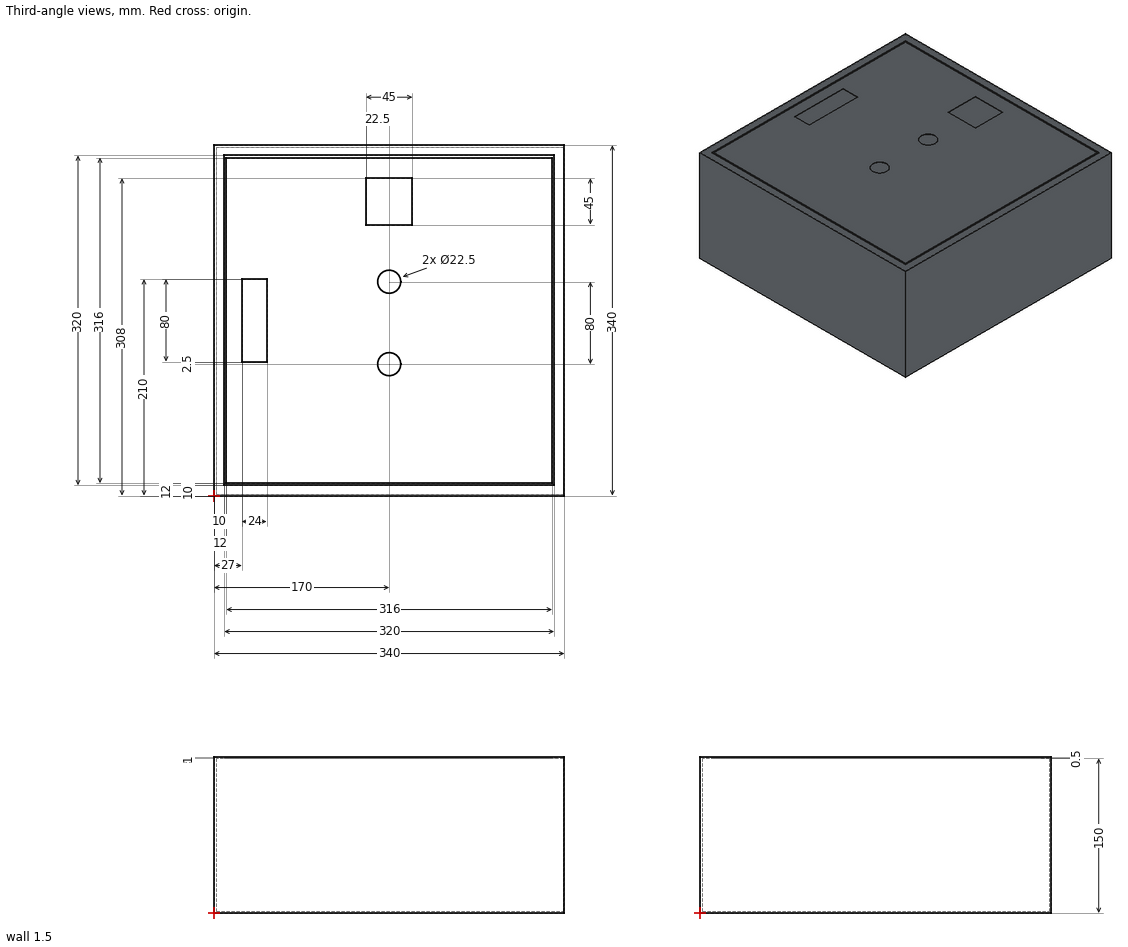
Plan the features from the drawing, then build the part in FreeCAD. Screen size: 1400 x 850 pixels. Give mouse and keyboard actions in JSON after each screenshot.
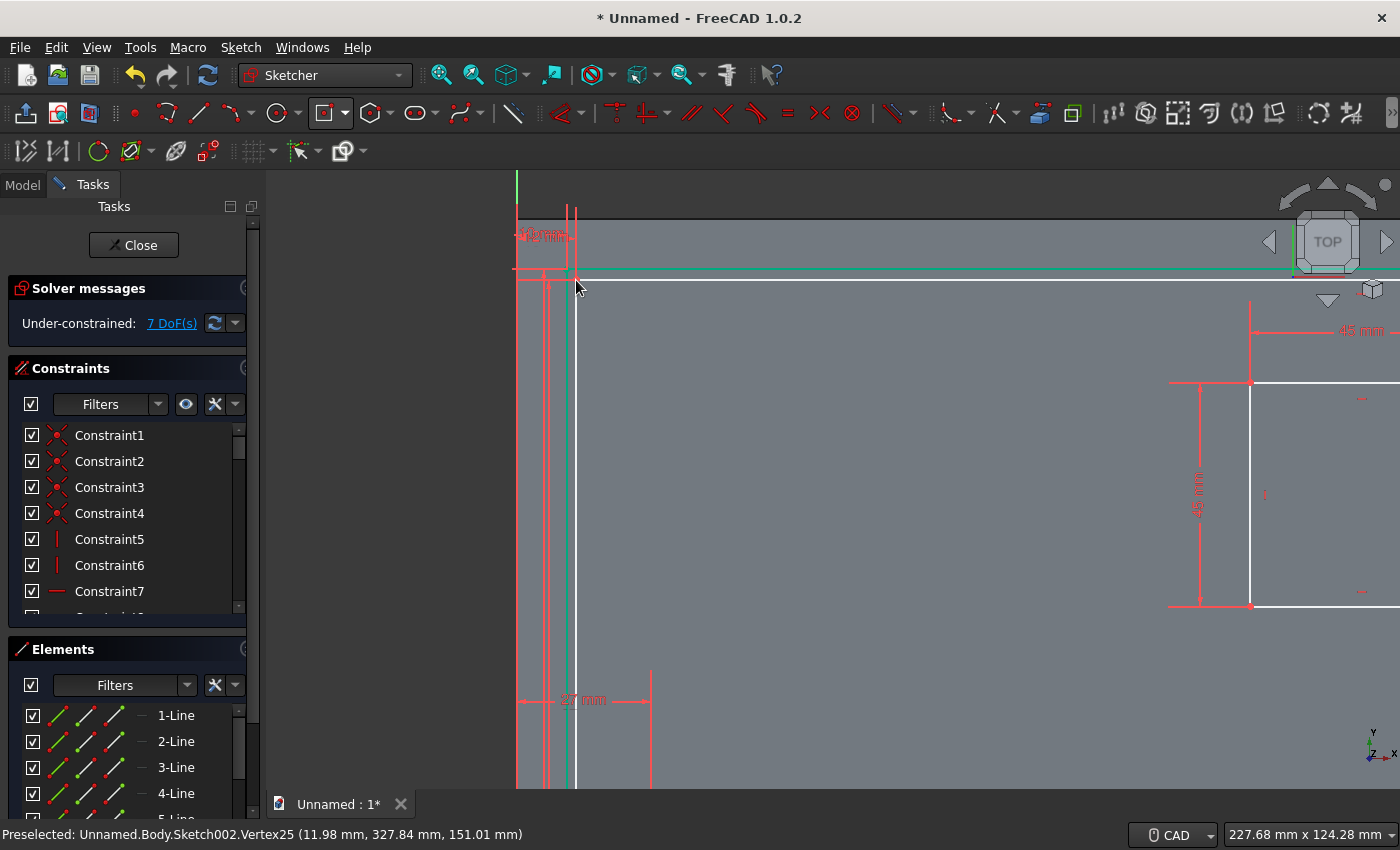
{"action": "scroll", "coordinate": [577, 279], "scroll_direction": "down", "scroll_amount": 7}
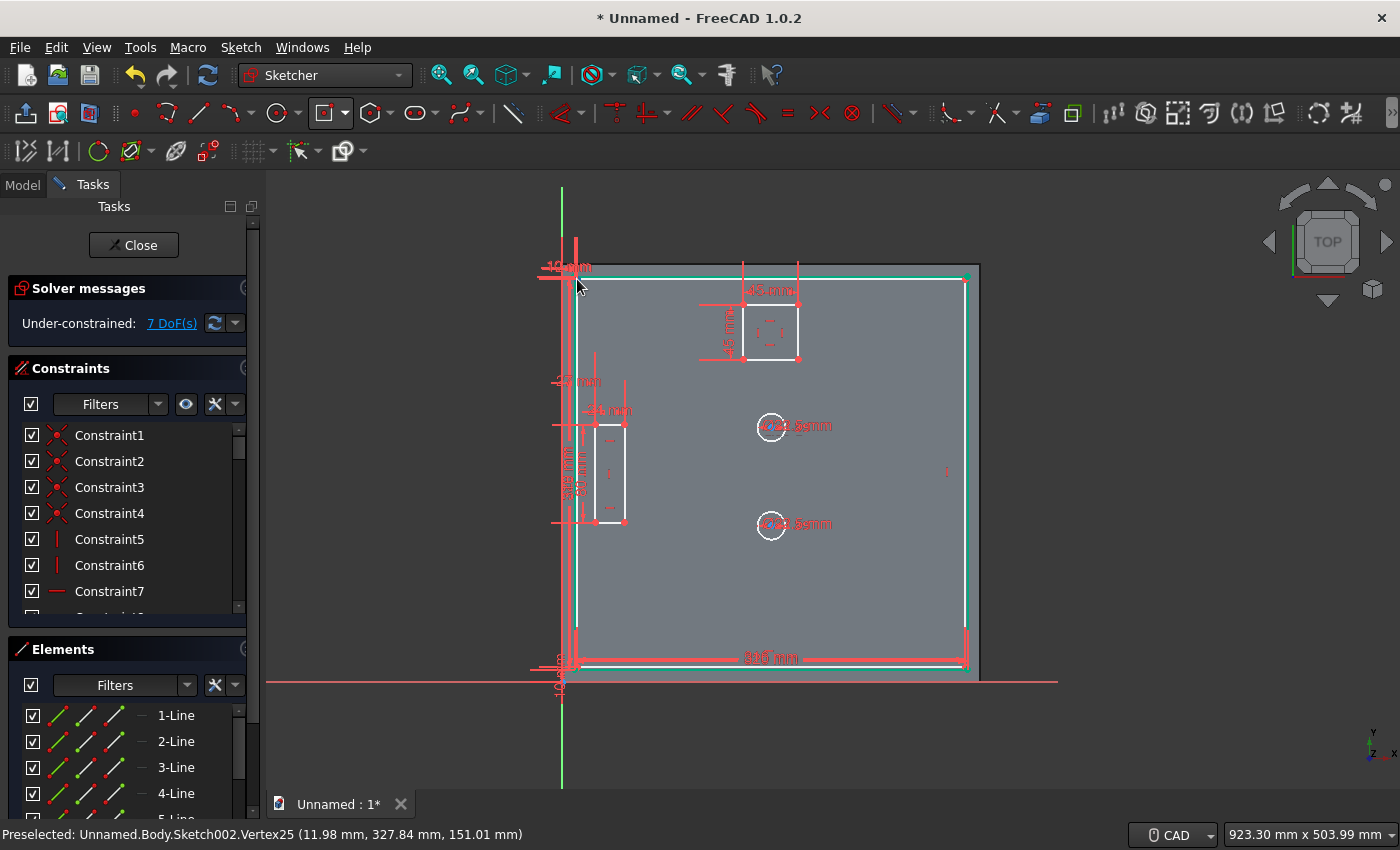
{"action": "scroll", "coordinate": [577, 667], "scroll_direction": "up", "scroll_amount": 7}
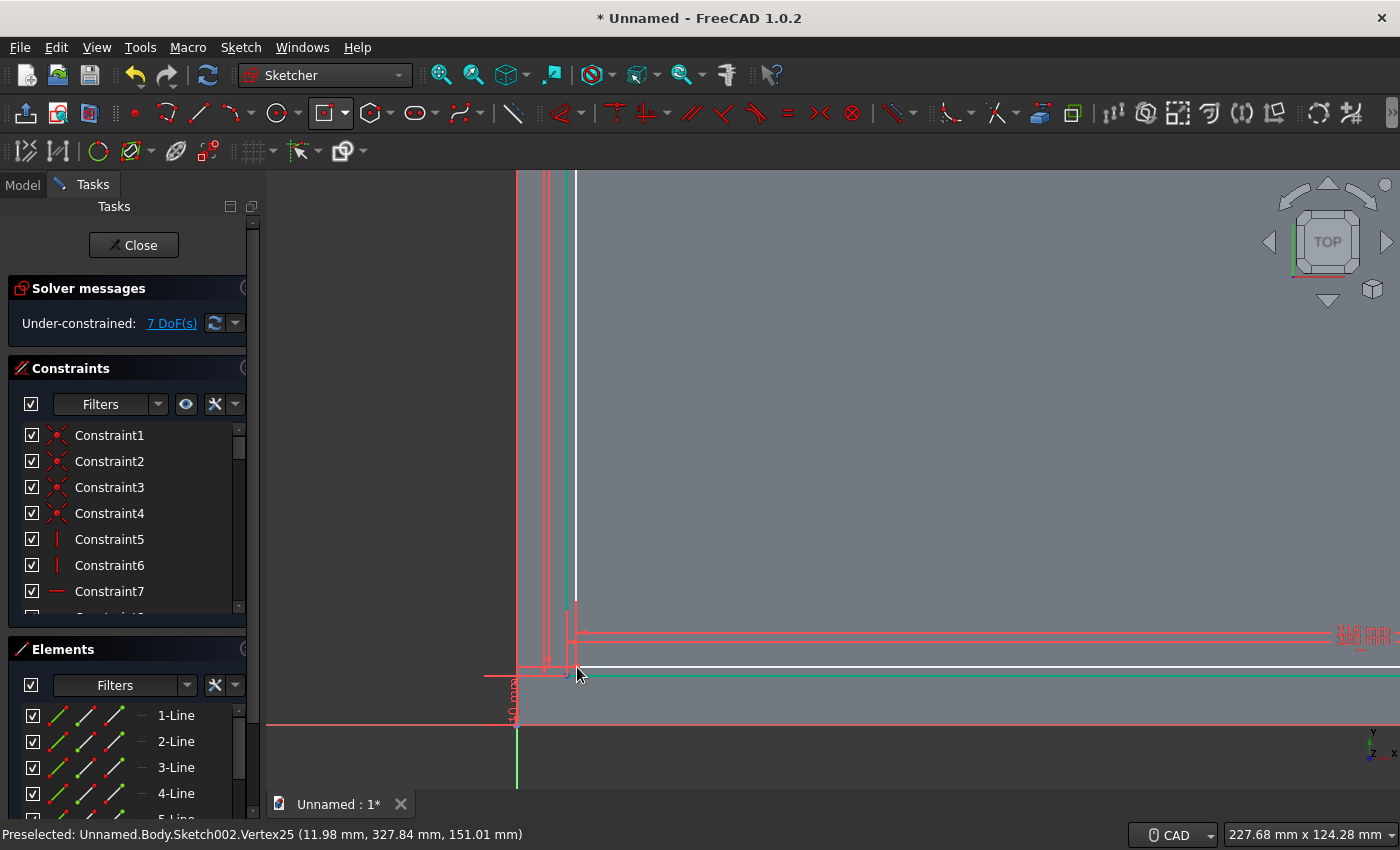
{"action": "left_click", "coordinate": [576, 667]}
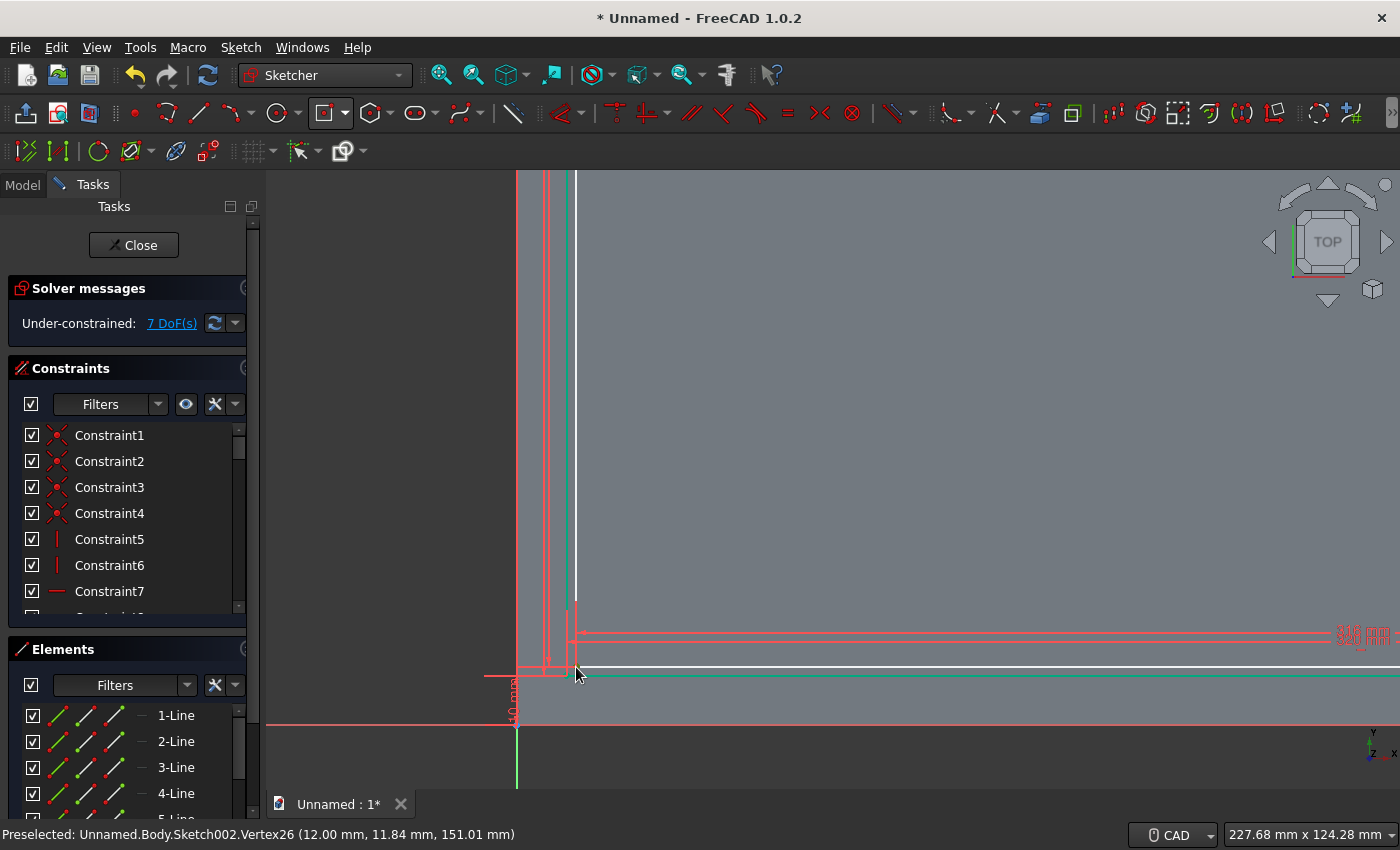
{"action": "key", "text": "i"}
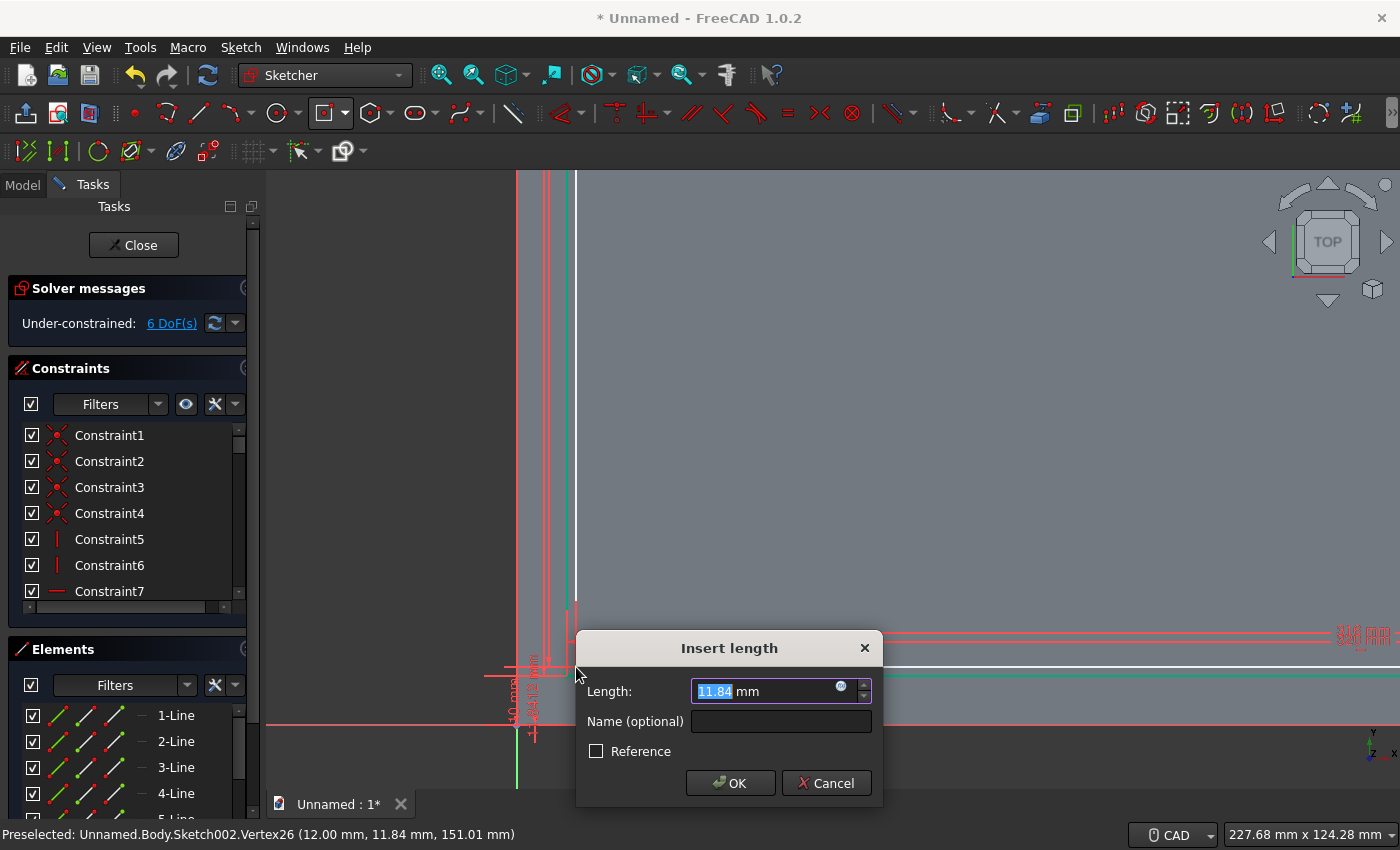
{"action": "type", "text": "12"}
{"action": "key", "text": "Return"}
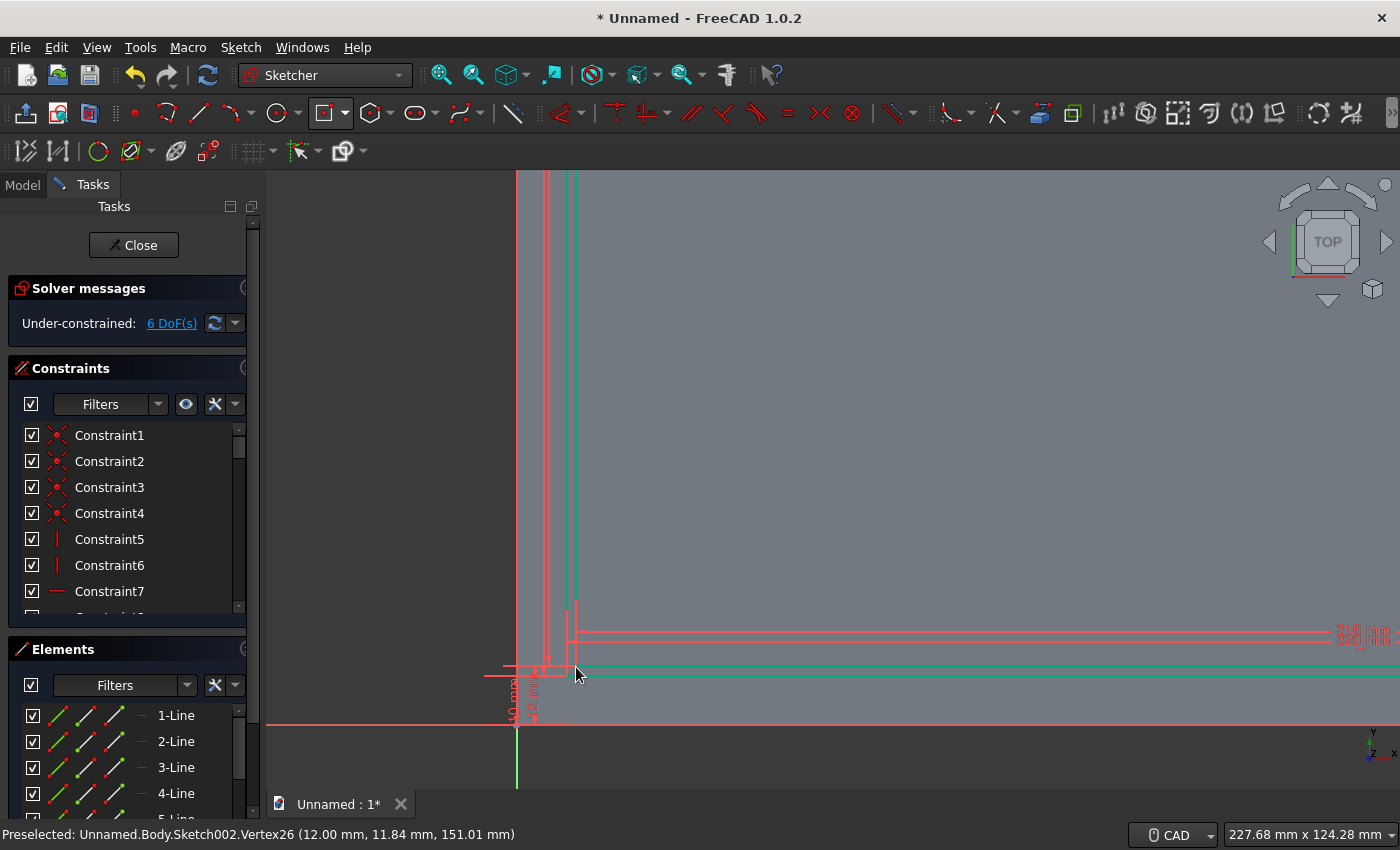
{"action": "scroll", "coordinate": [577, 668], "scroll_direction": "down", "scroll_amount": 7}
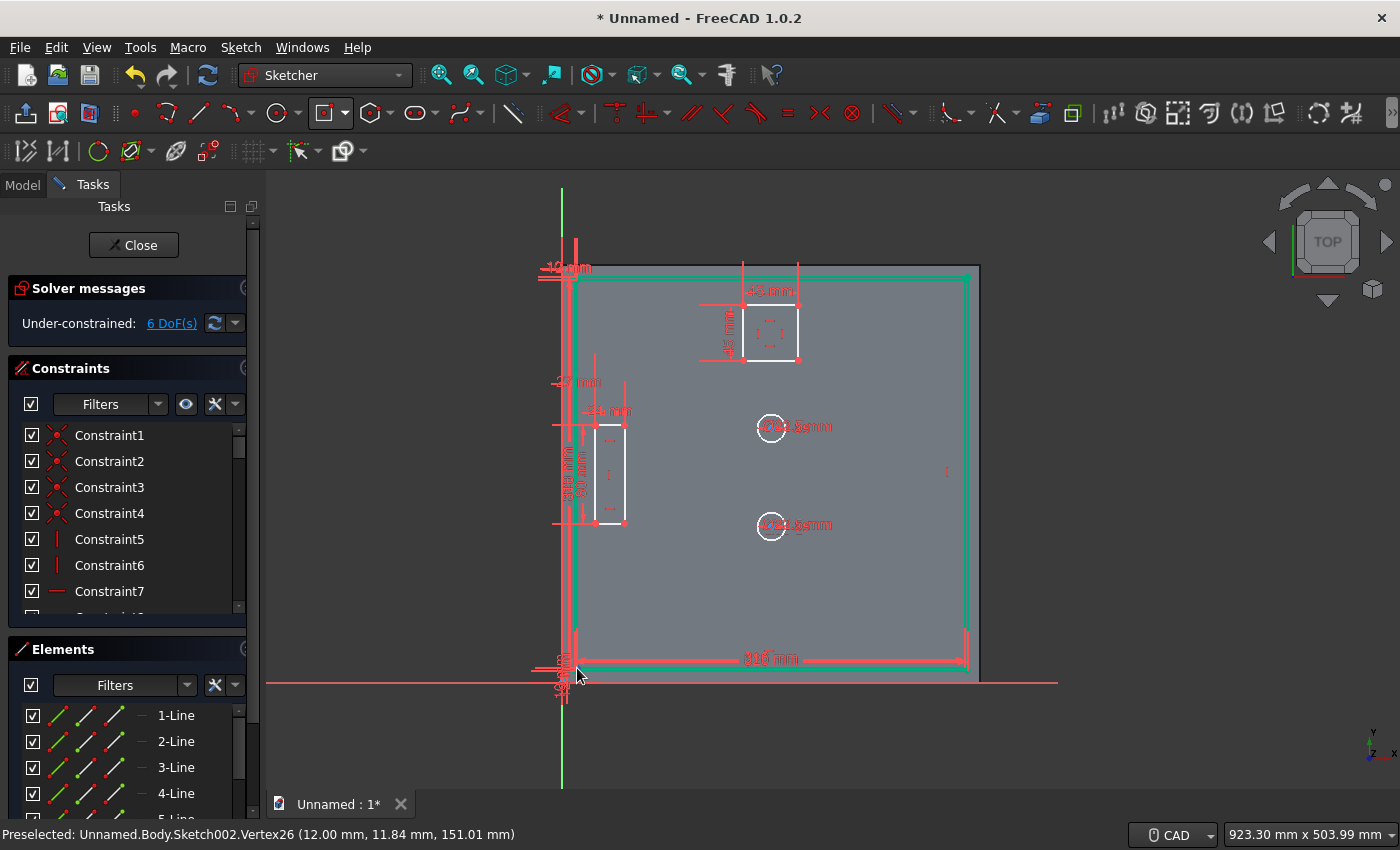
{"action": "left_click", "coordinate": [771, 428]}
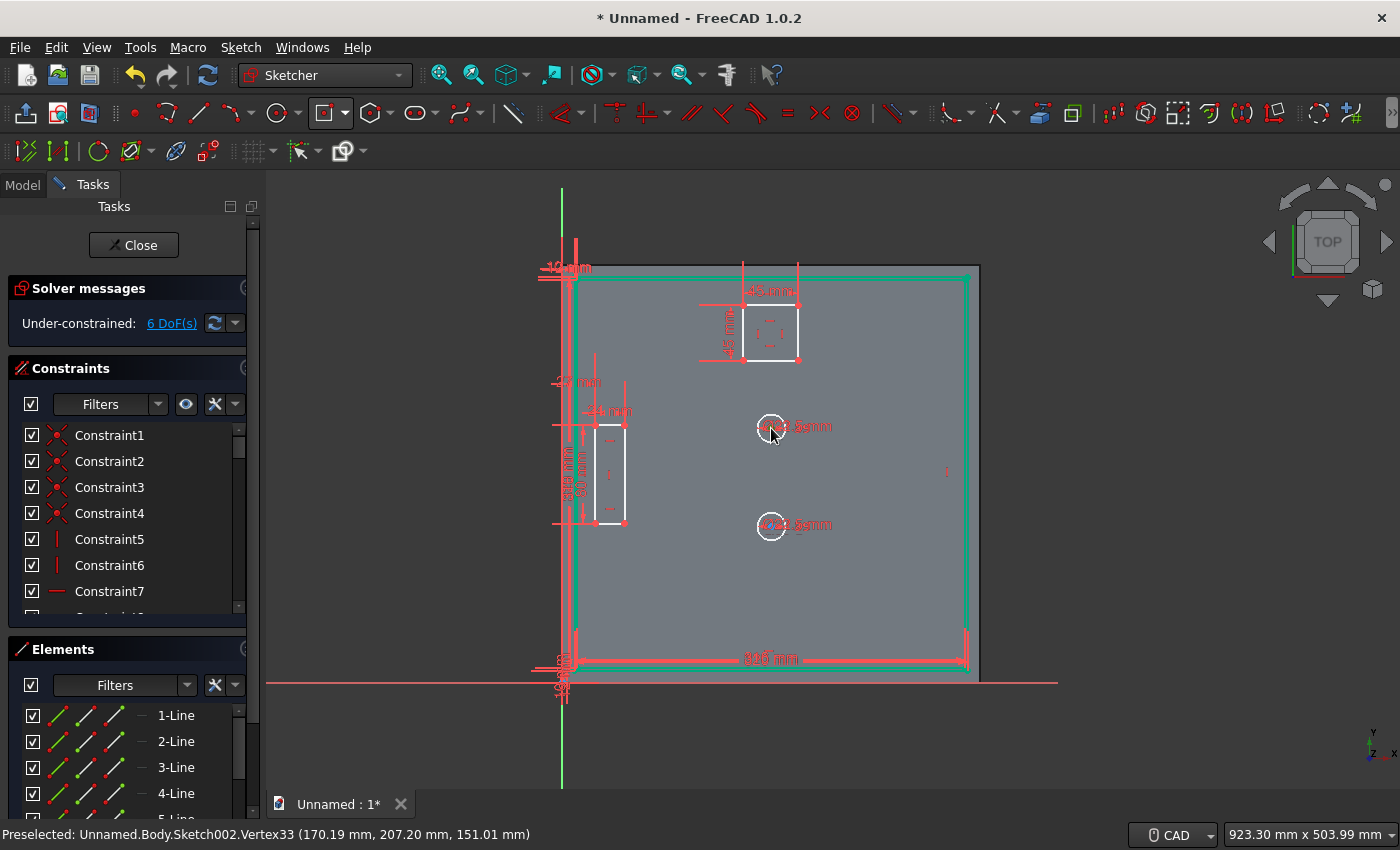
{"action": "left_click", "coordinate": [584, 114]}